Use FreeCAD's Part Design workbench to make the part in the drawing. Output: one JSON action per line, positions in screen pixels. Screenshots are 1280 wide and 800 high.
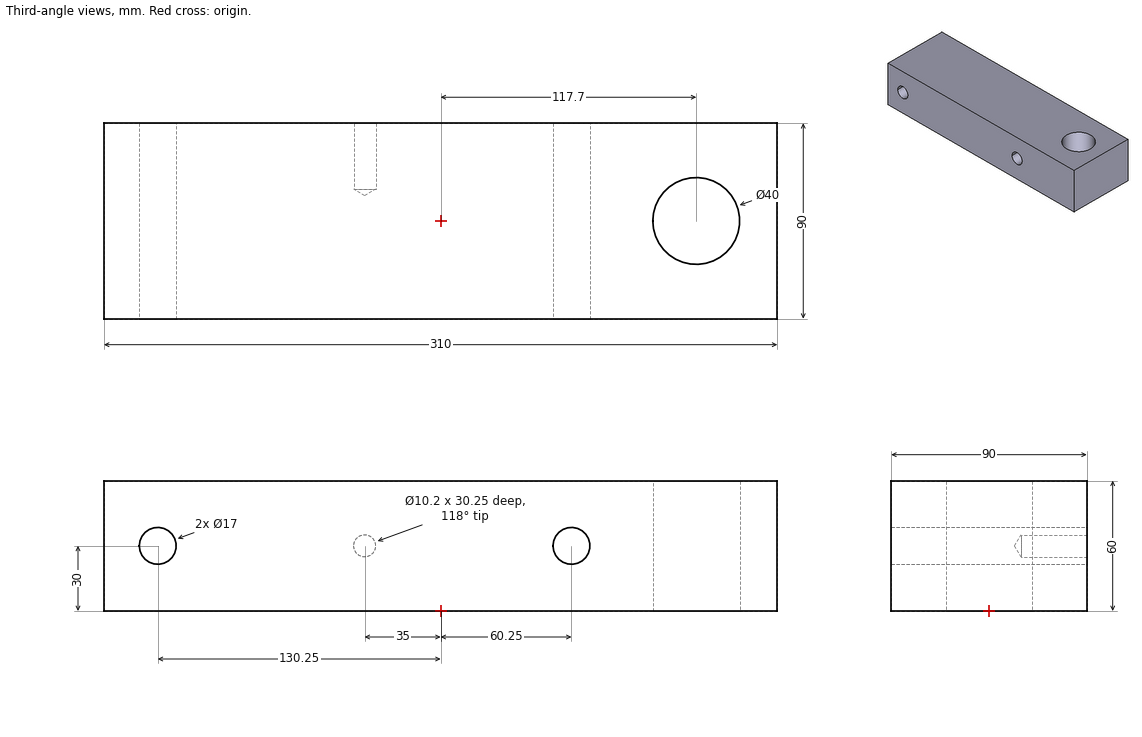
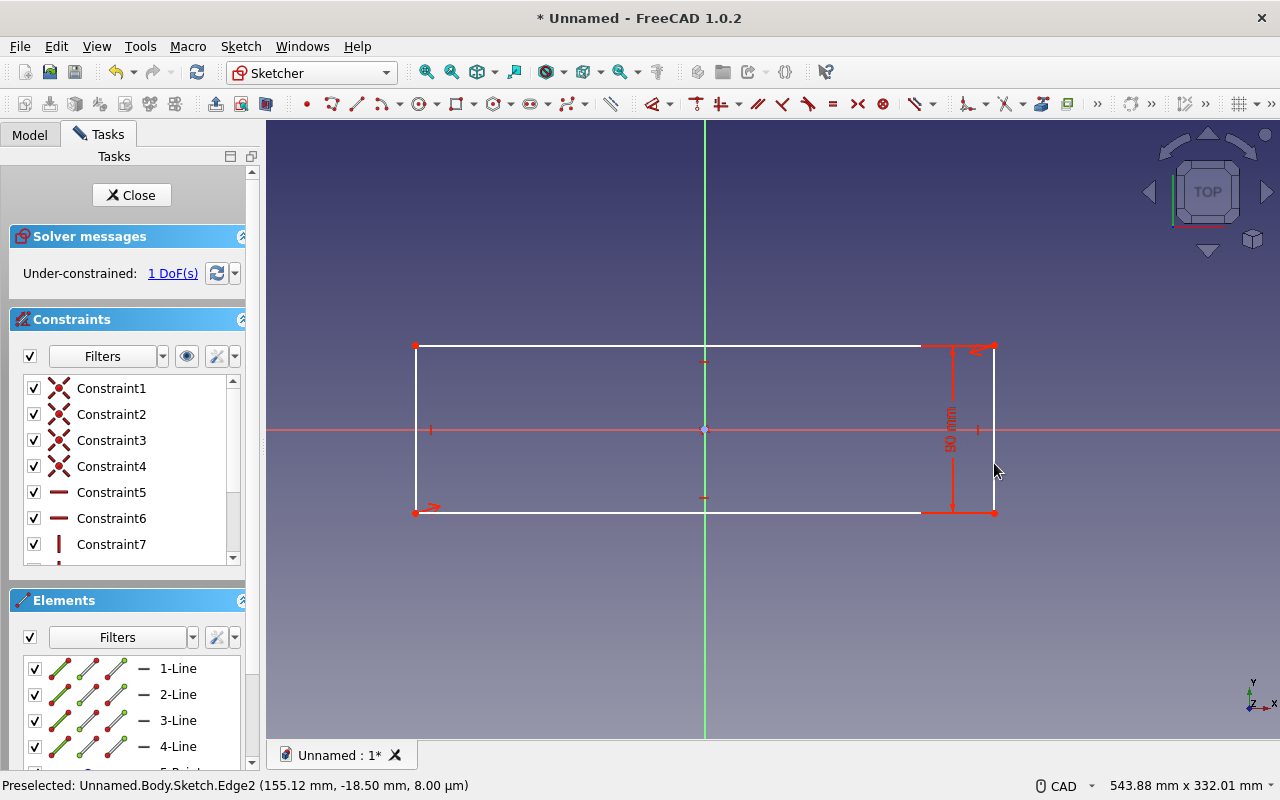
{"action": "left_click", "coordinate": [589, 513]}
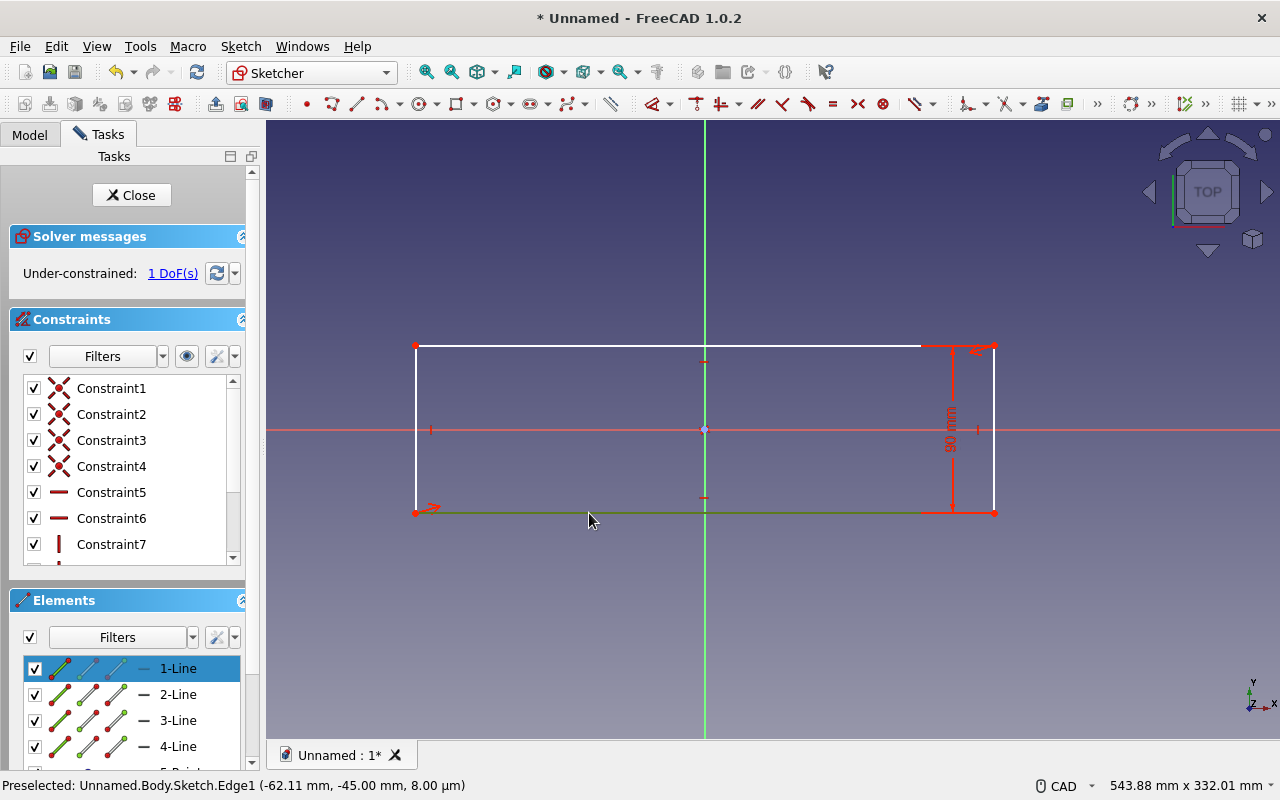
{"action": "left_click", "coordinate": [670, 104]}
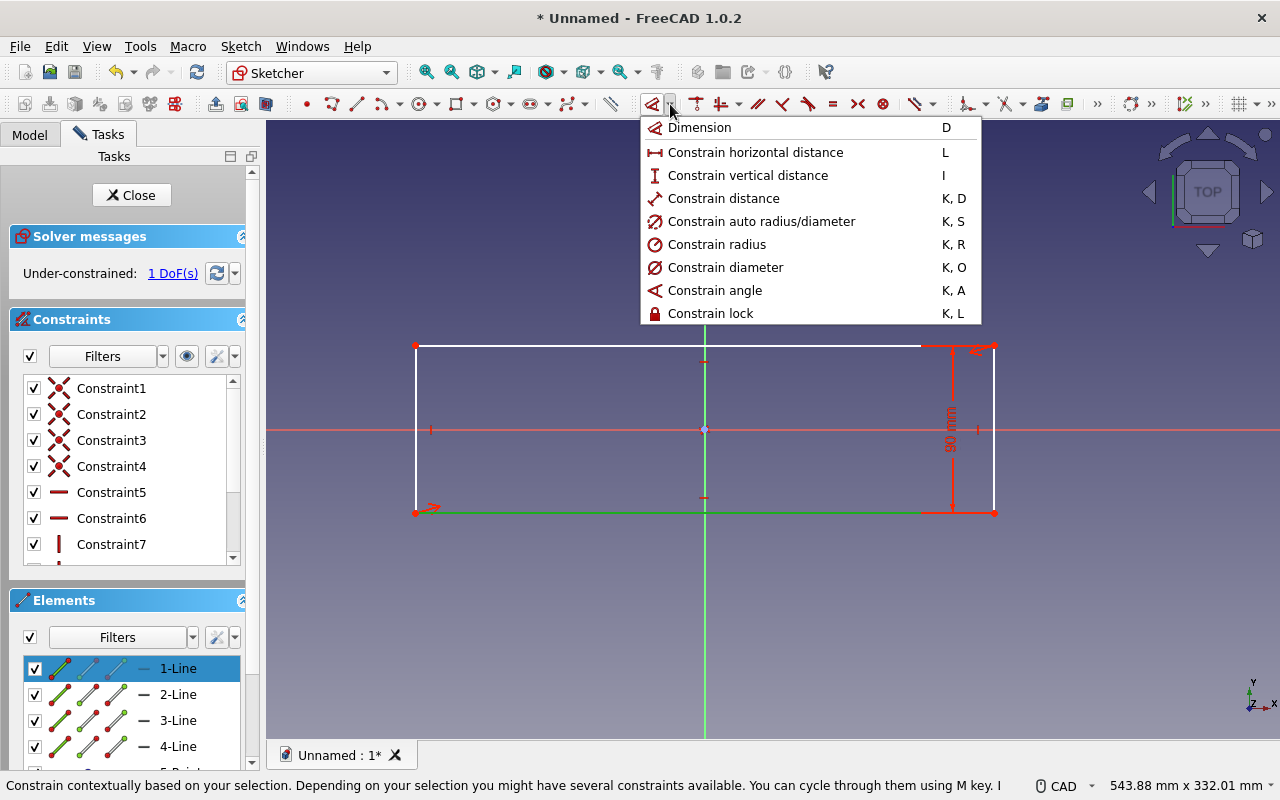
{"action": "left_click", "coordinate": [811, 152]}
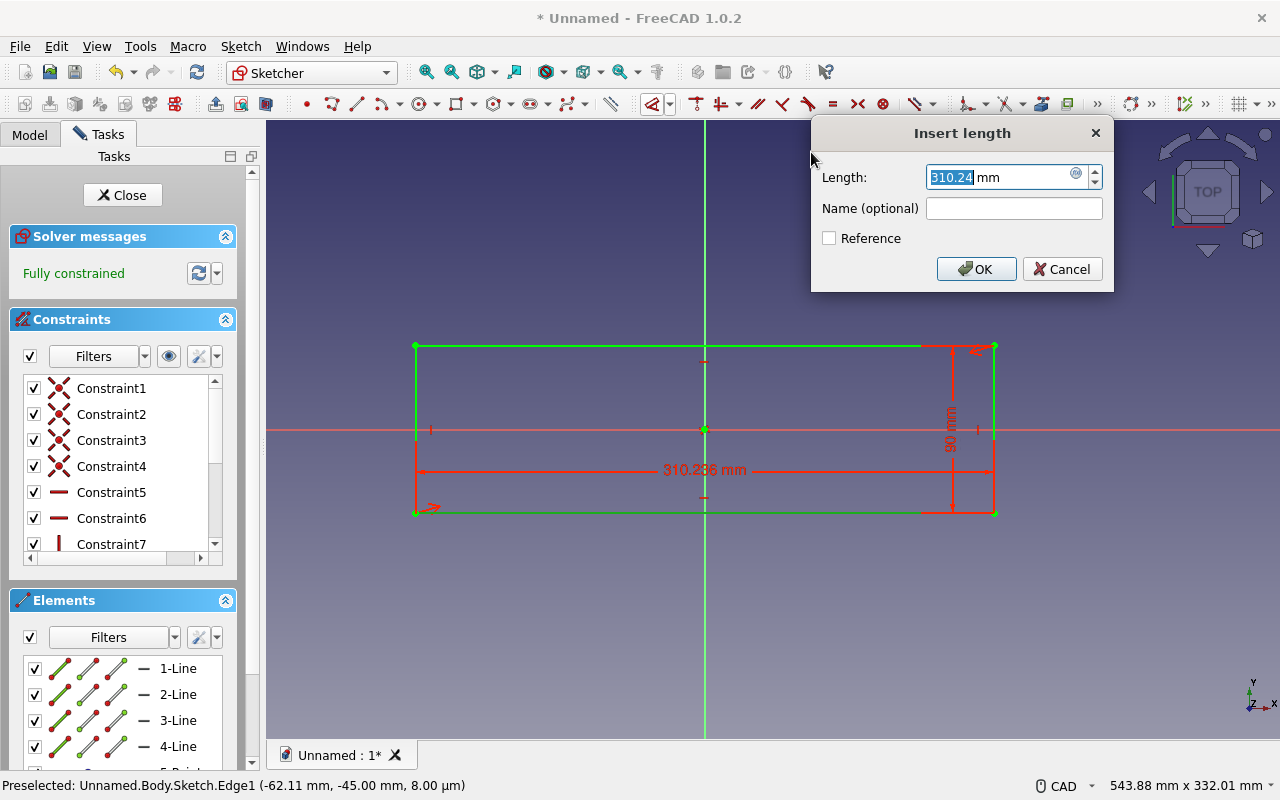
{"action": "type", "text": "310"}
{"action": "key", "text": "Return"}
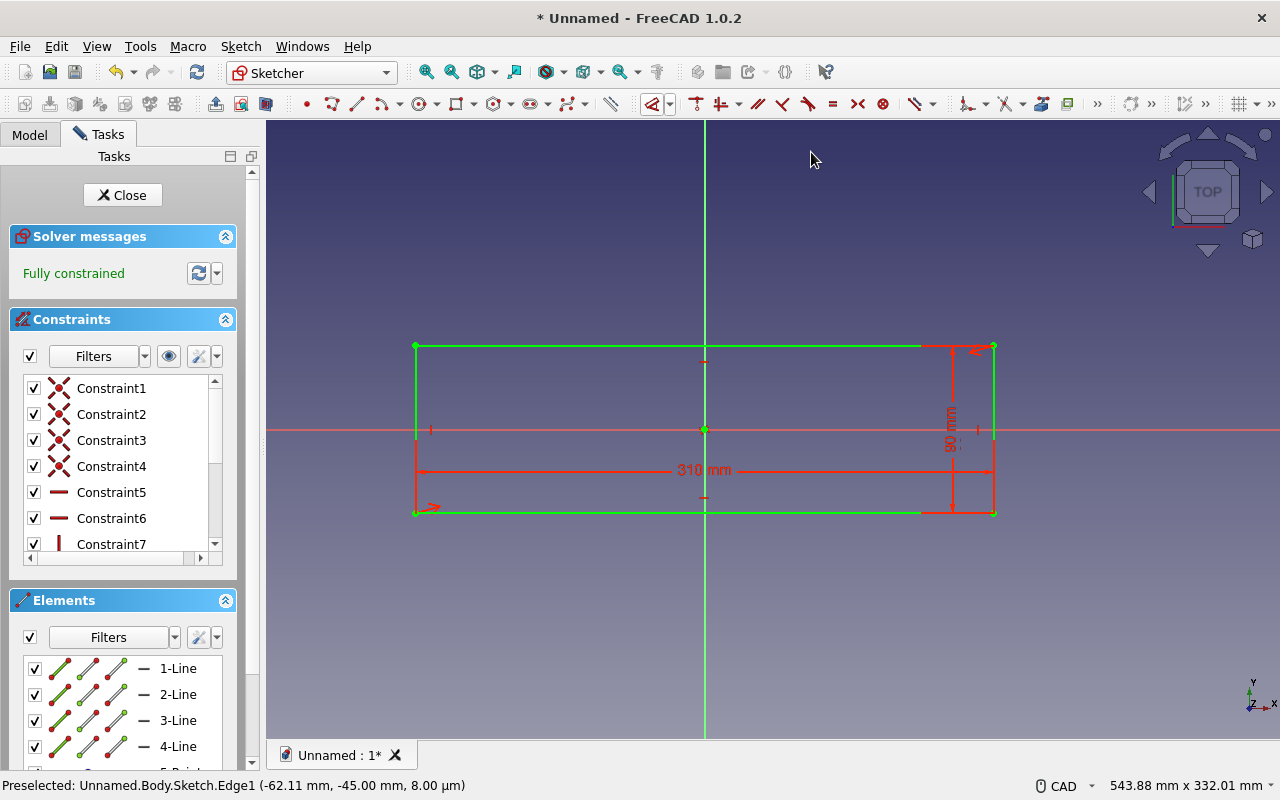
{"action": "left_click", "coordinate": [123, 195]}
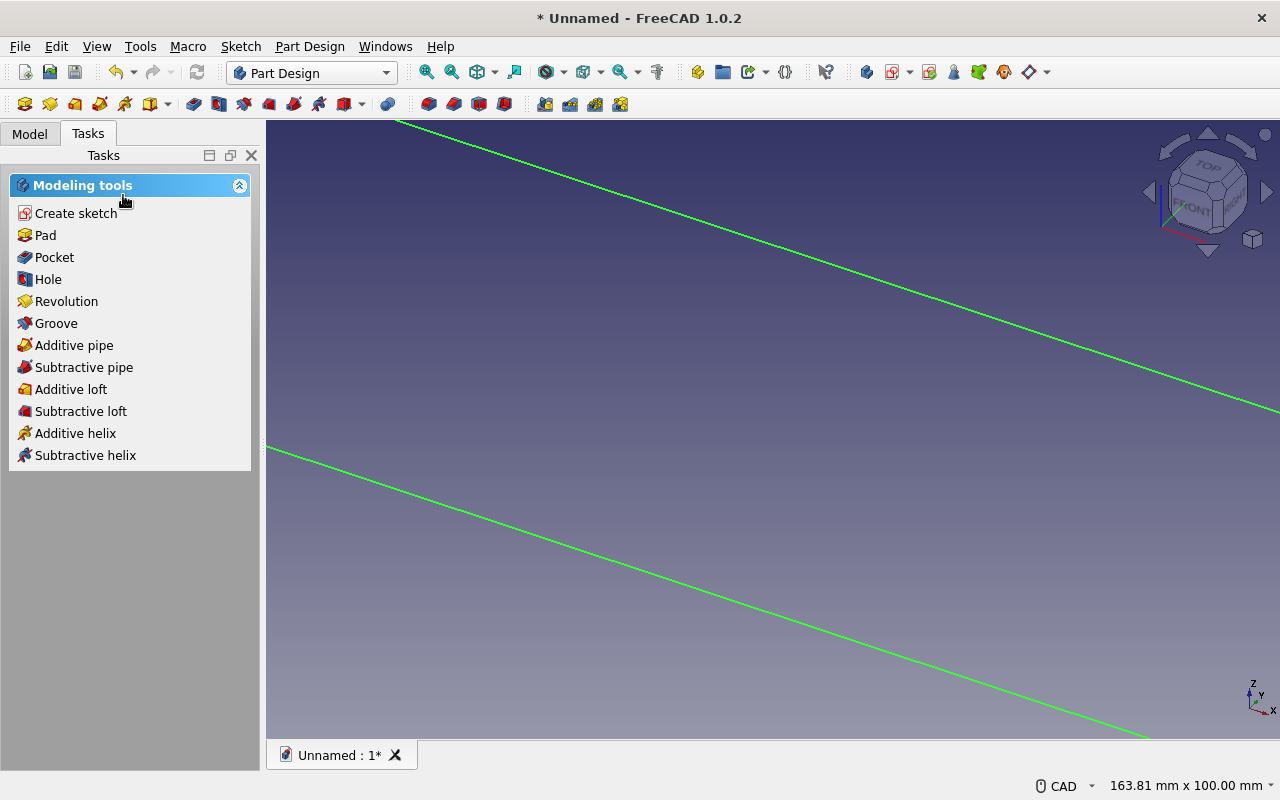
{"action": "left_click", "coordinate": [25, 104]}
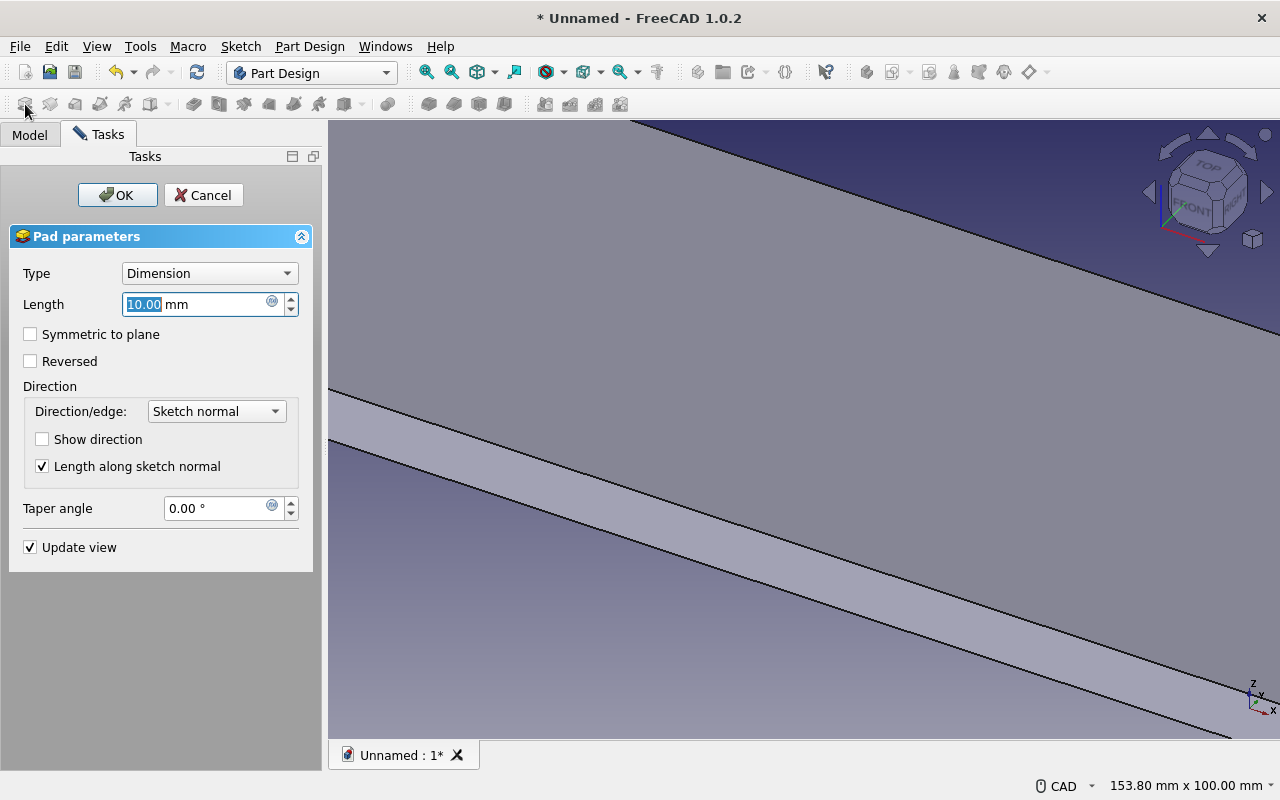
{"action": "type", "text": "60"}
{"action": "key", "text": "Tab"}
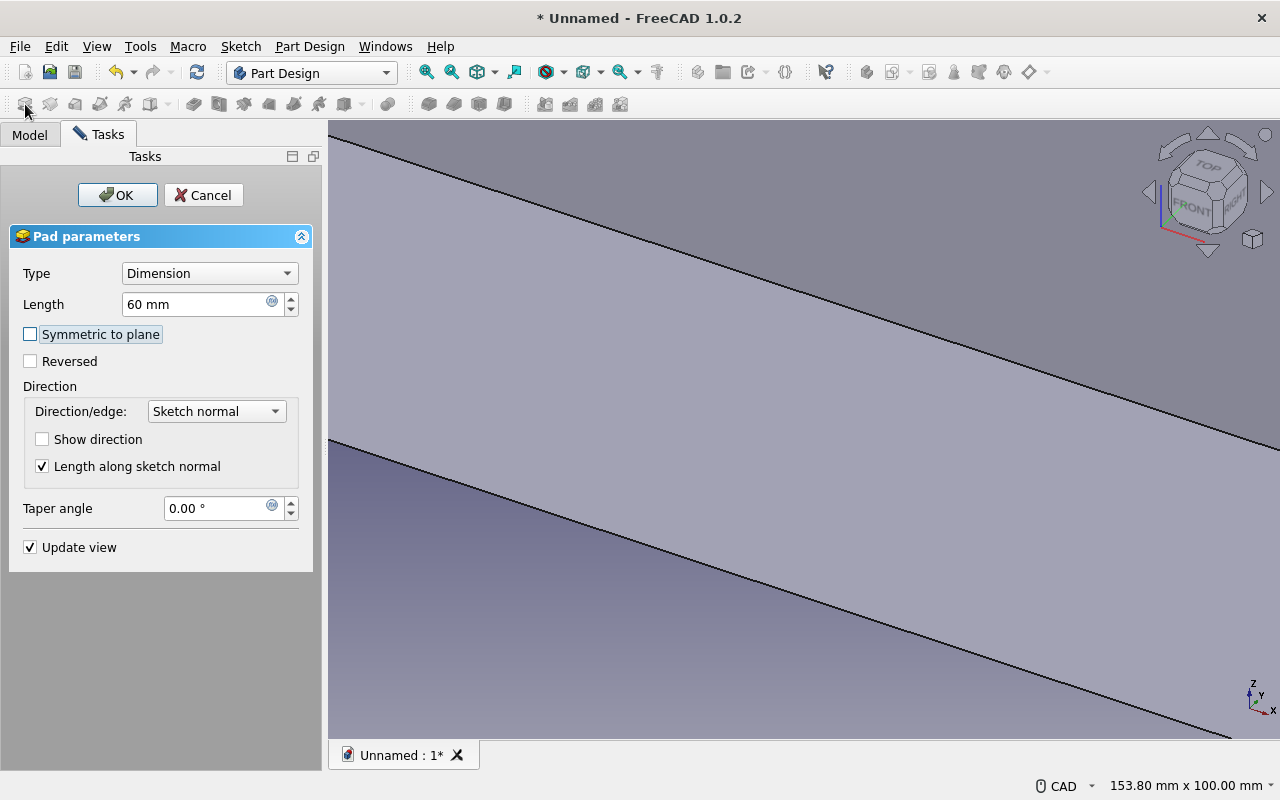
{"action": "left_click", "coordinate": [118, 195]}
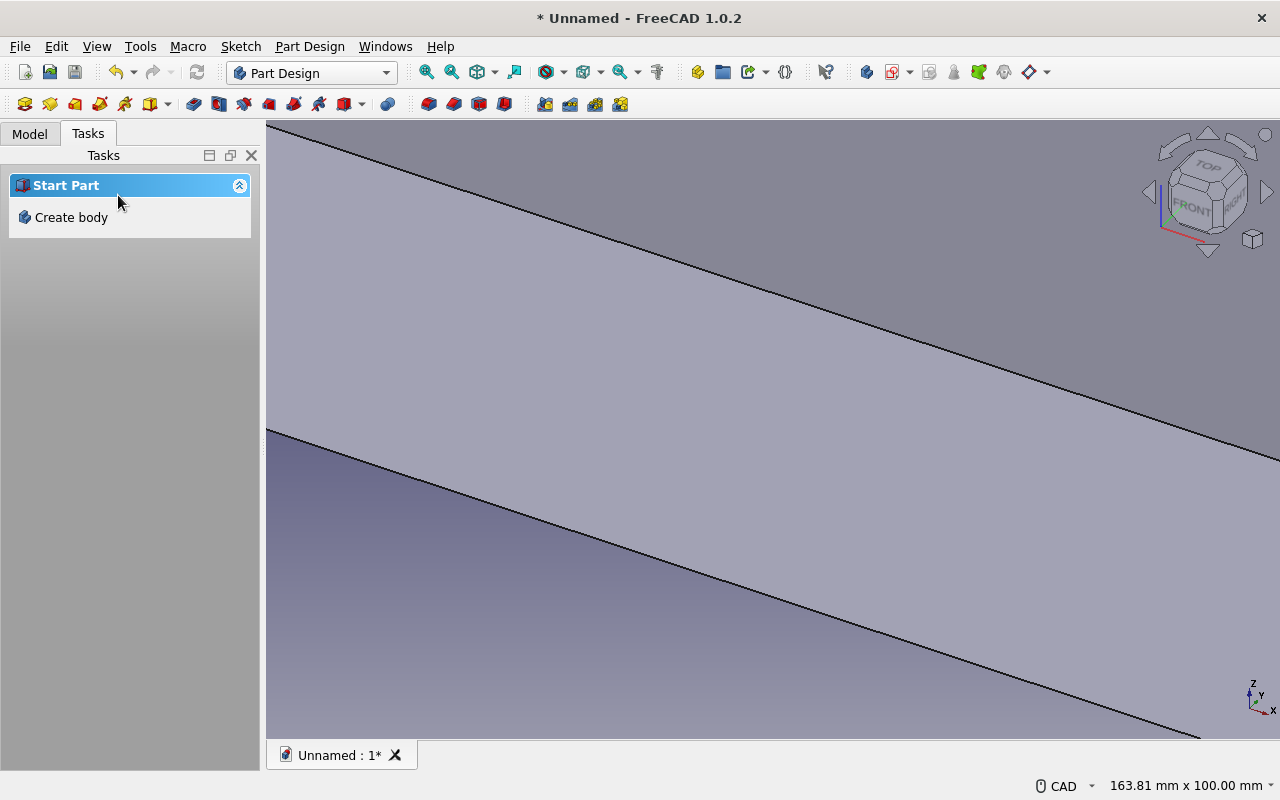
{"action": "key", "text": "v f"}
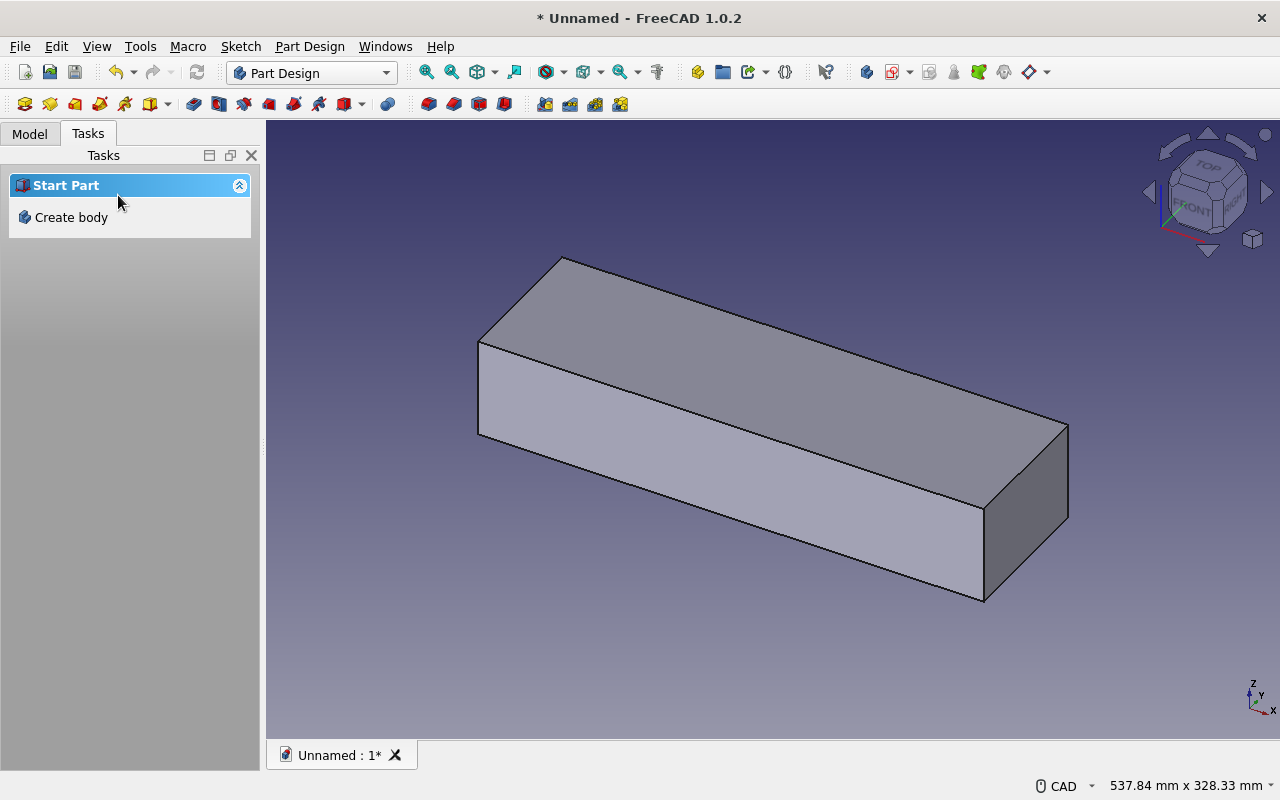
{"action": "key", "text": "4"}